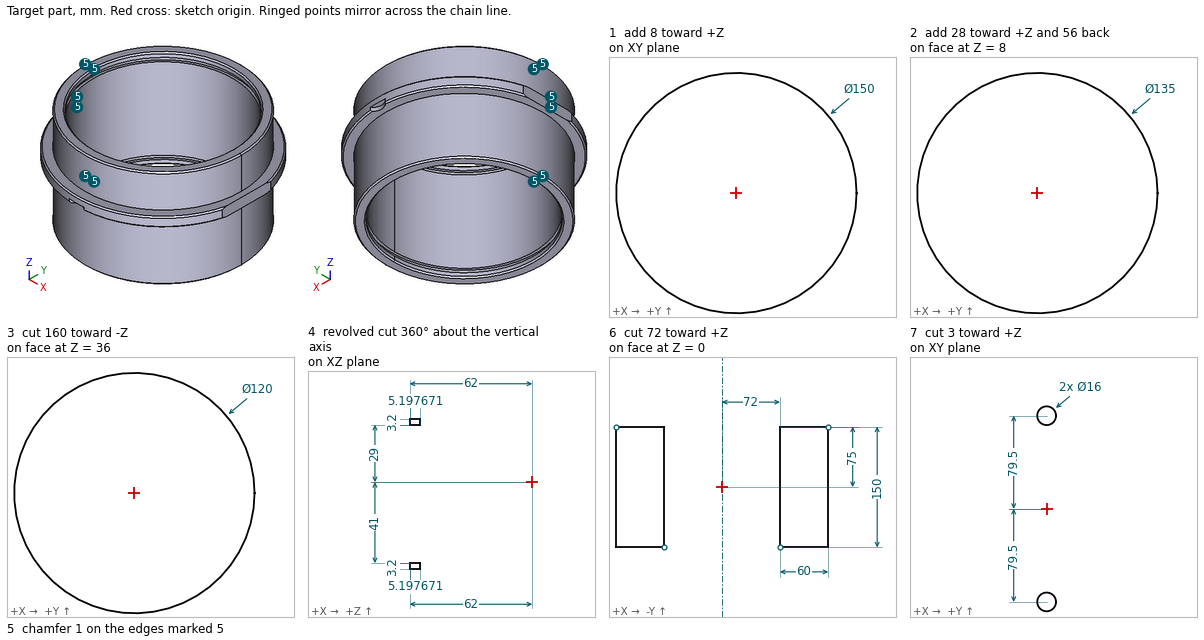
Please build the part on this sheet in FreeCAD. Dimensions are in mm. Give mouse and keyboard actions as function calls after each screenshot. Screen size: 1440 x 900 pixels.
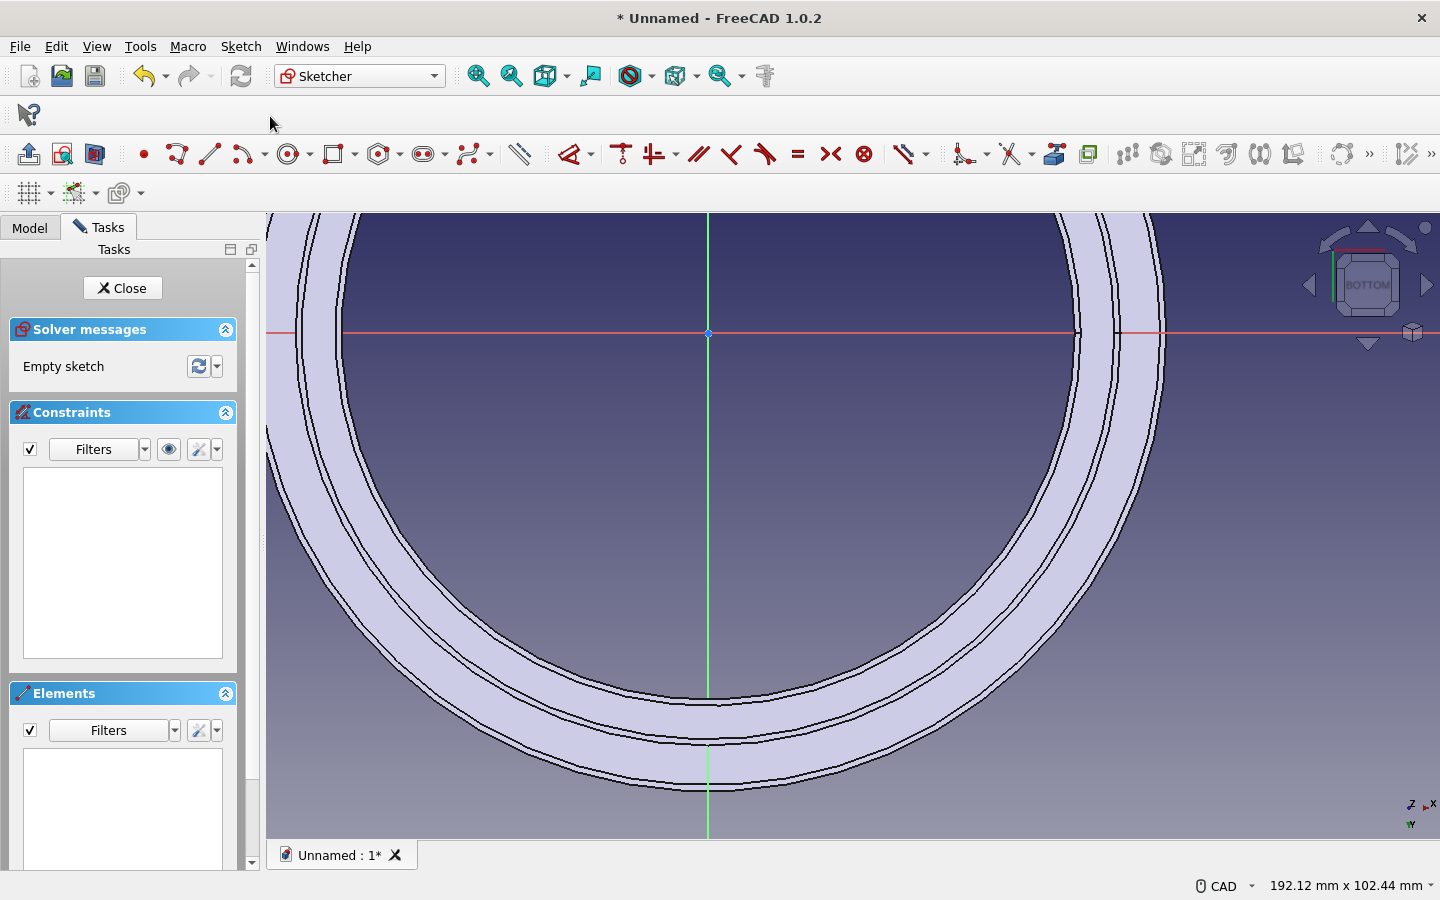
key(q)
key(s)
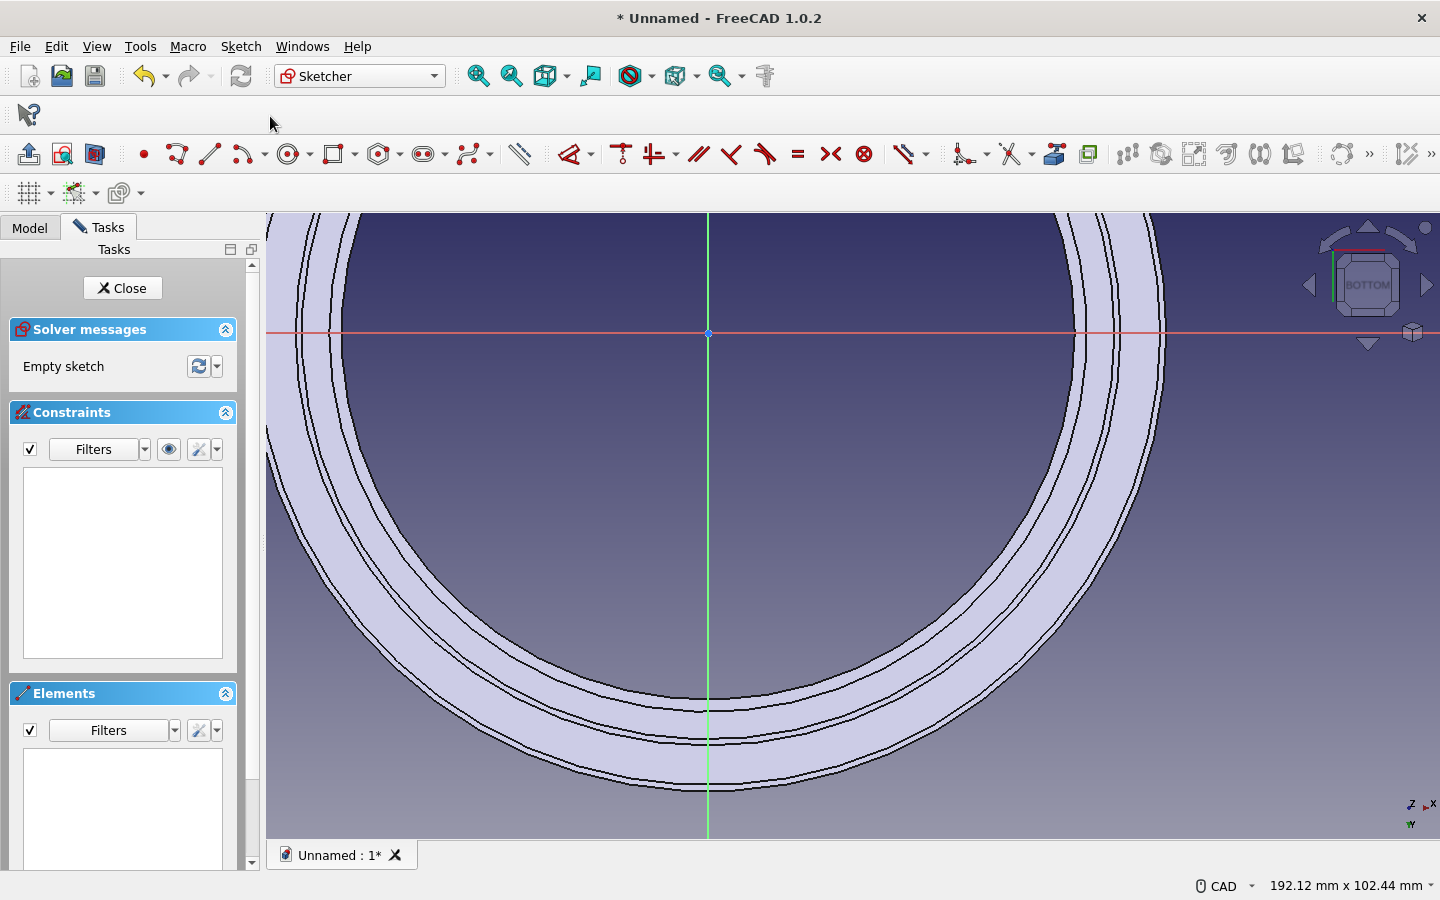
scroll(847, 683, down, 4)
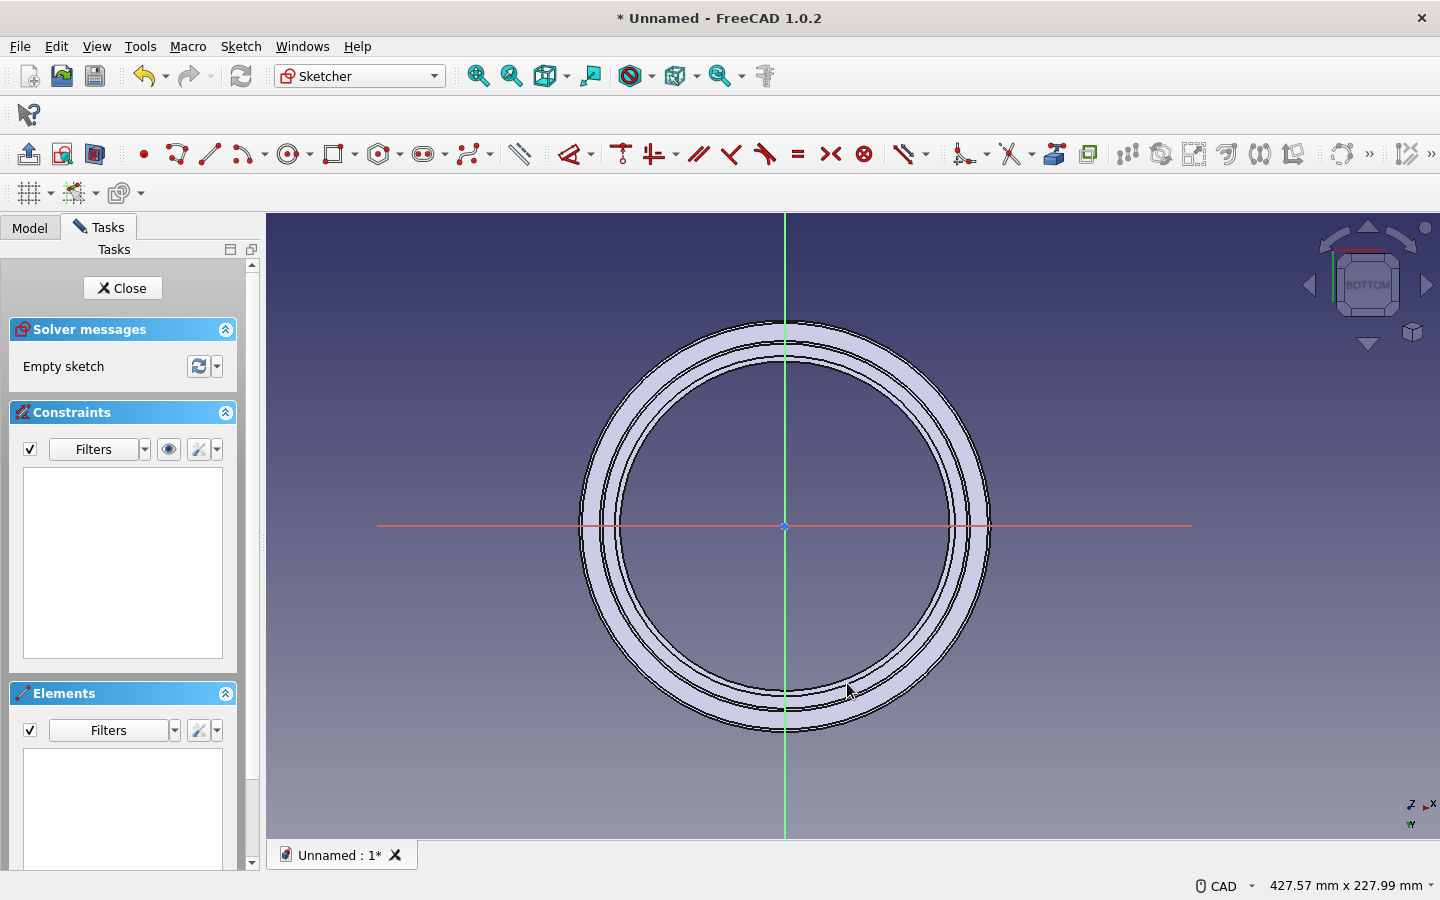
key(g)
key(r)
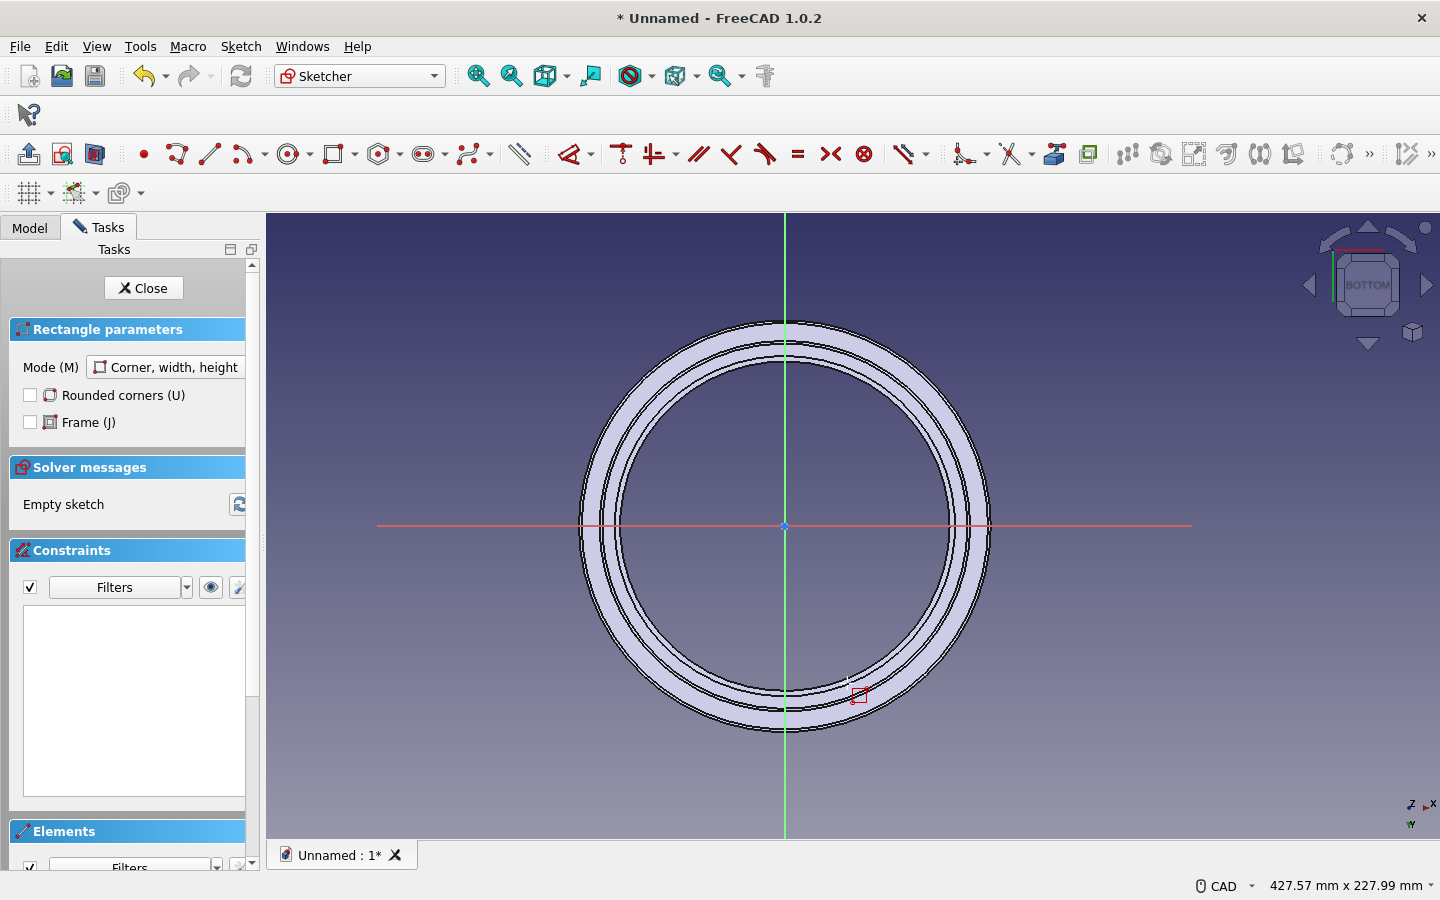
click(983, 320)
click(1147, 732)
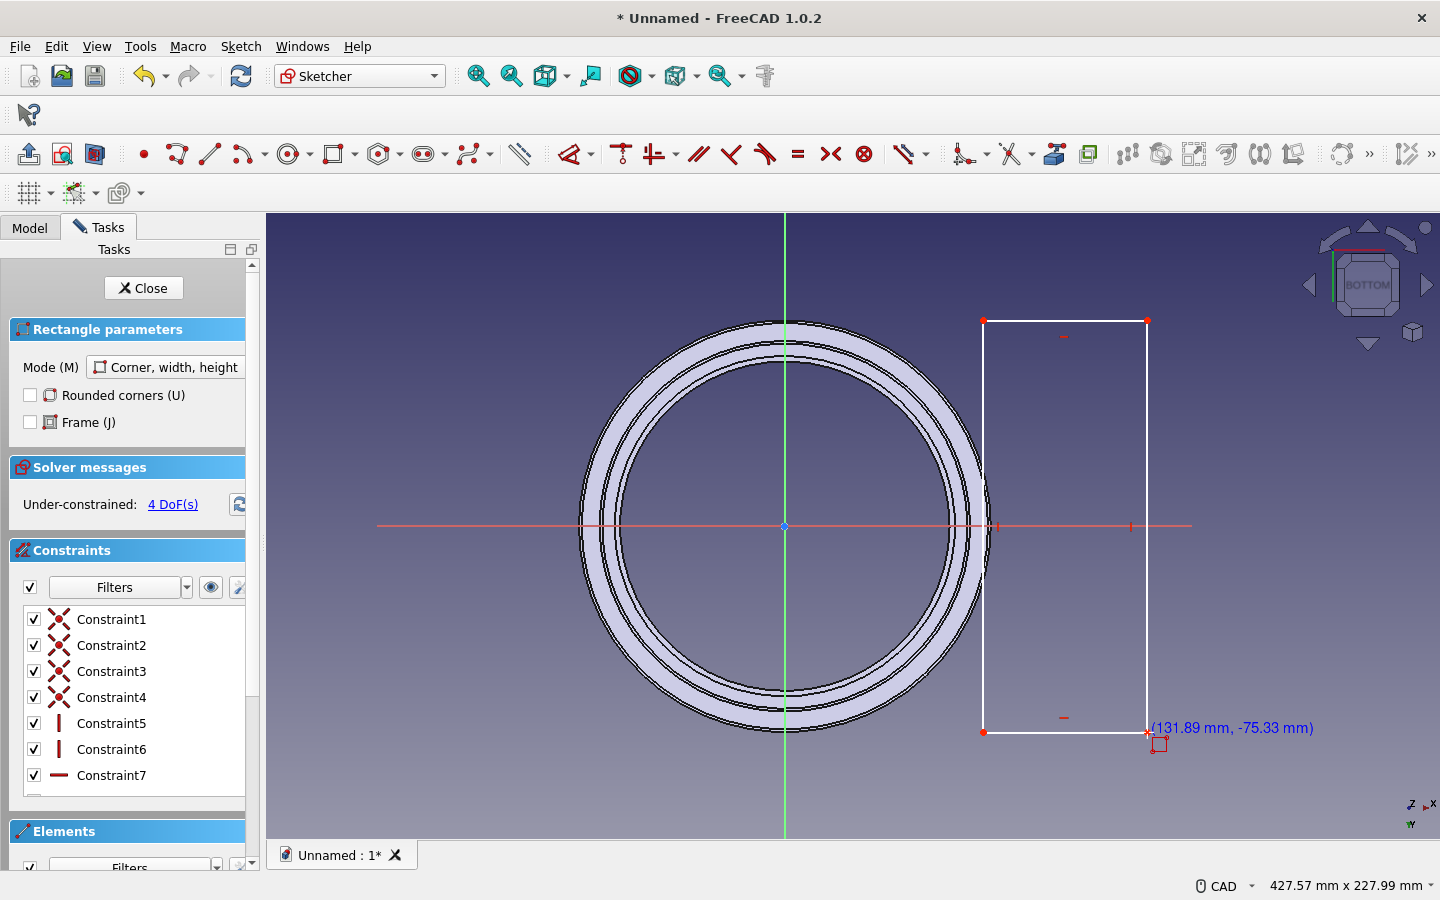
click(422, 320)
click(587, 732)
key(Escape)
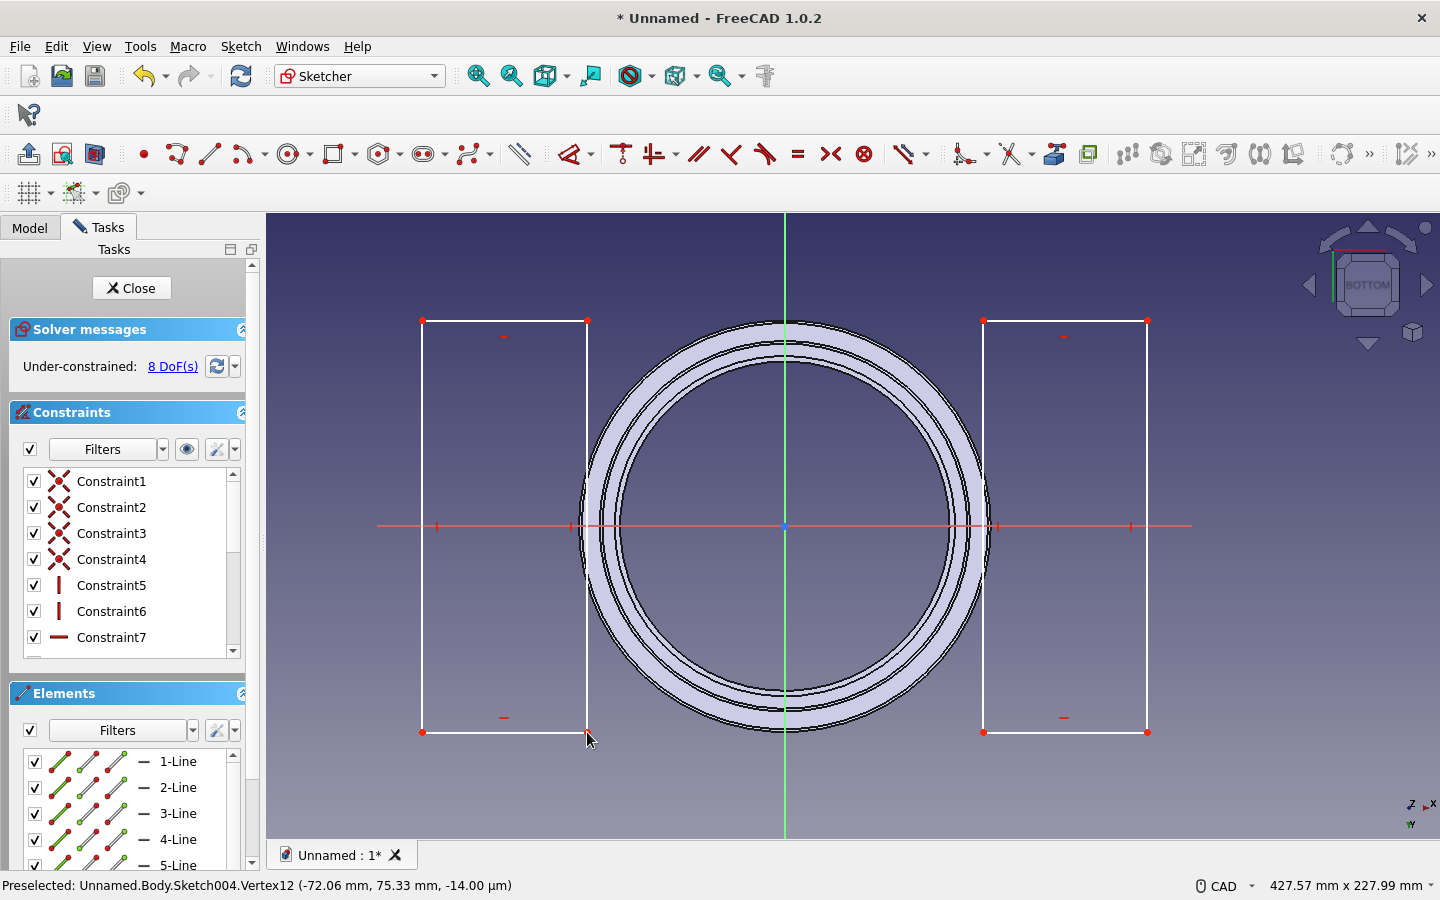
click(1147, 321)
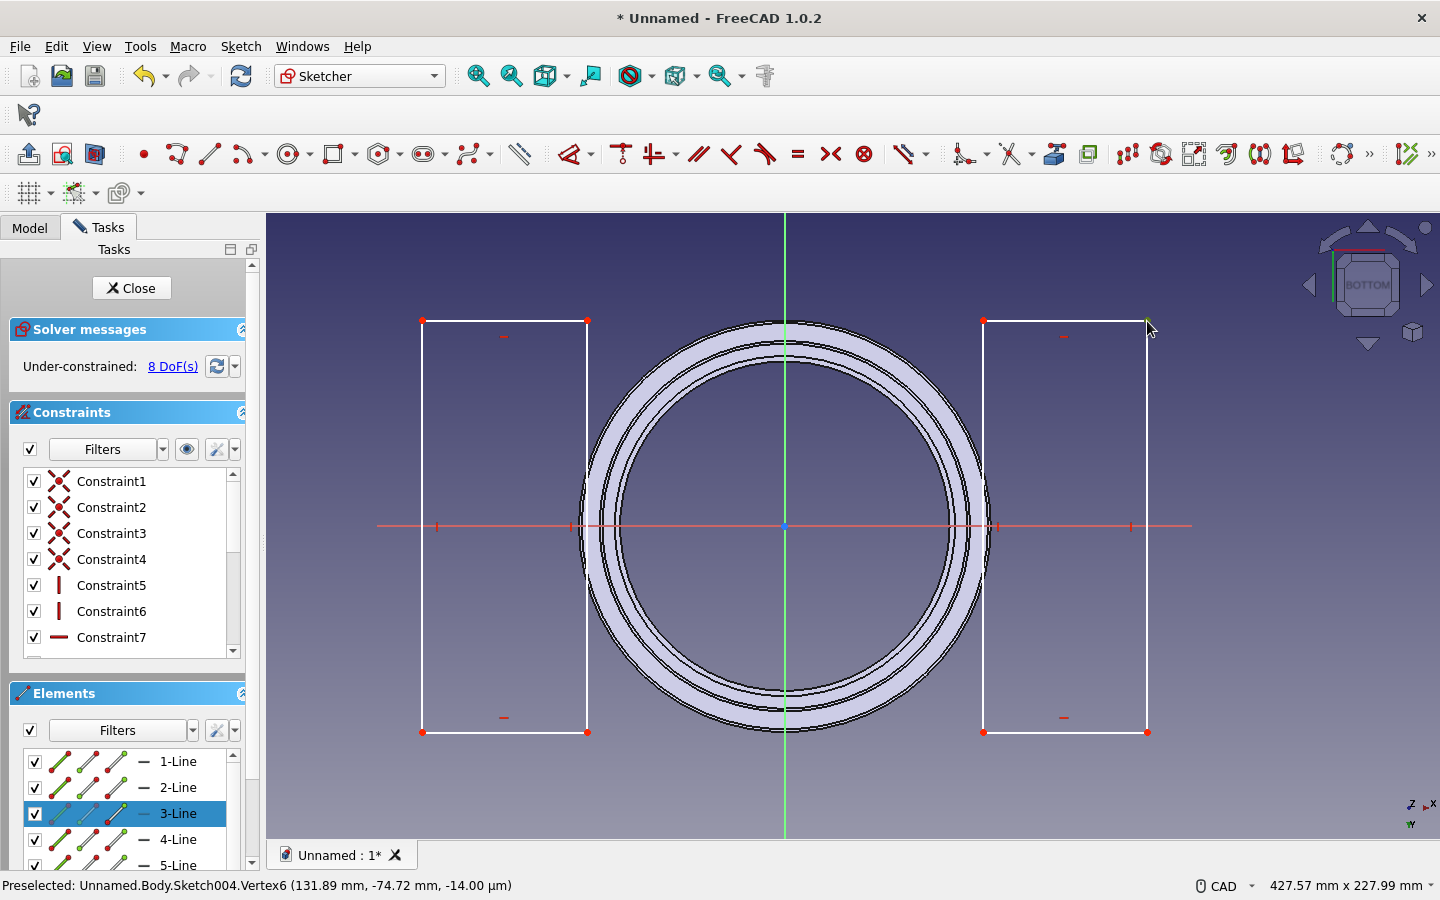
click(422, 321)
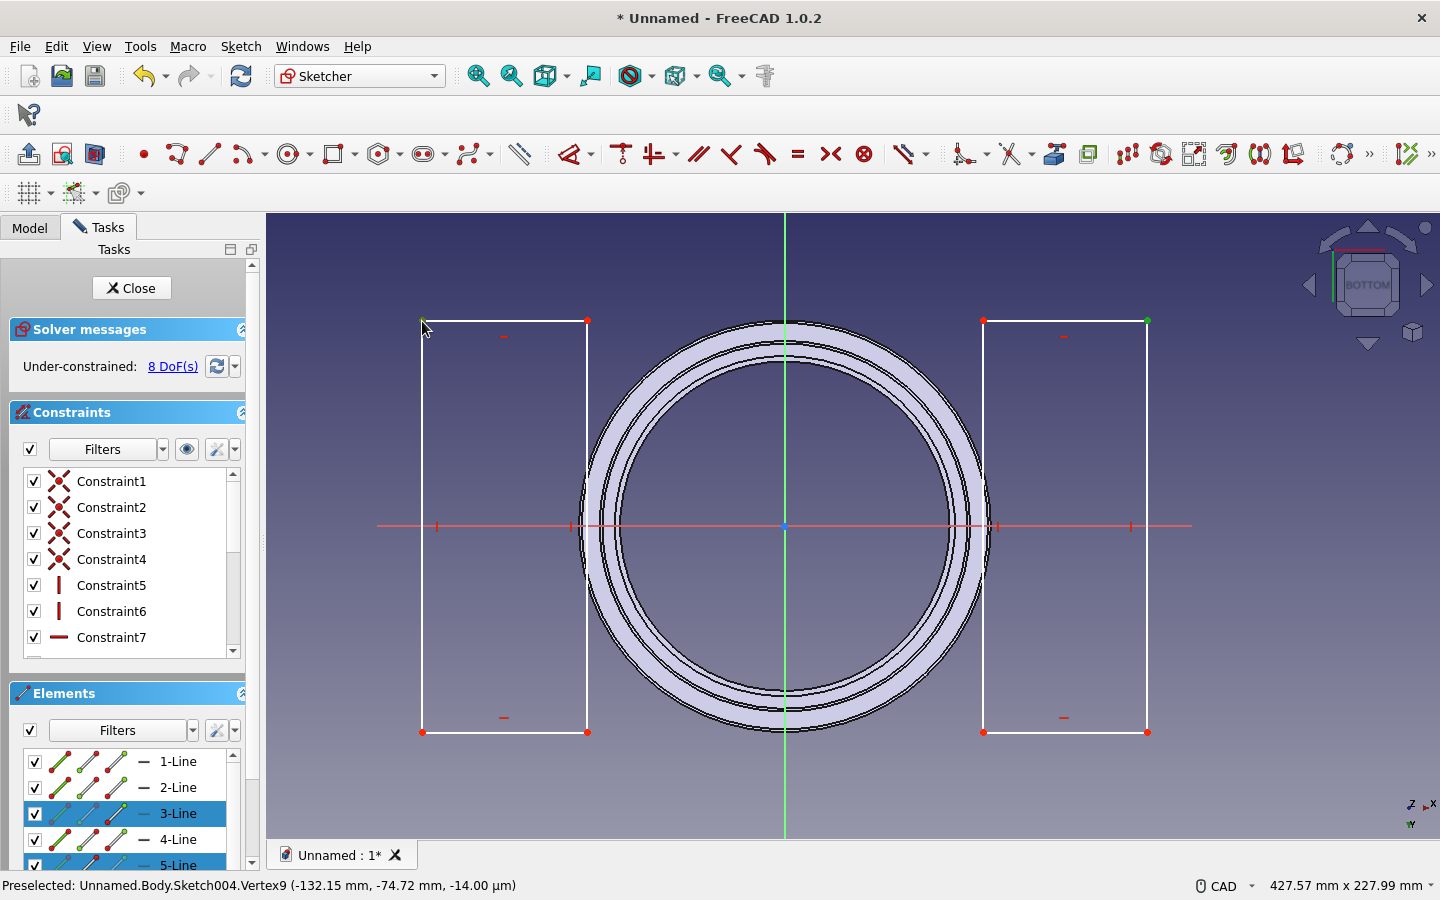
click(785, 770)